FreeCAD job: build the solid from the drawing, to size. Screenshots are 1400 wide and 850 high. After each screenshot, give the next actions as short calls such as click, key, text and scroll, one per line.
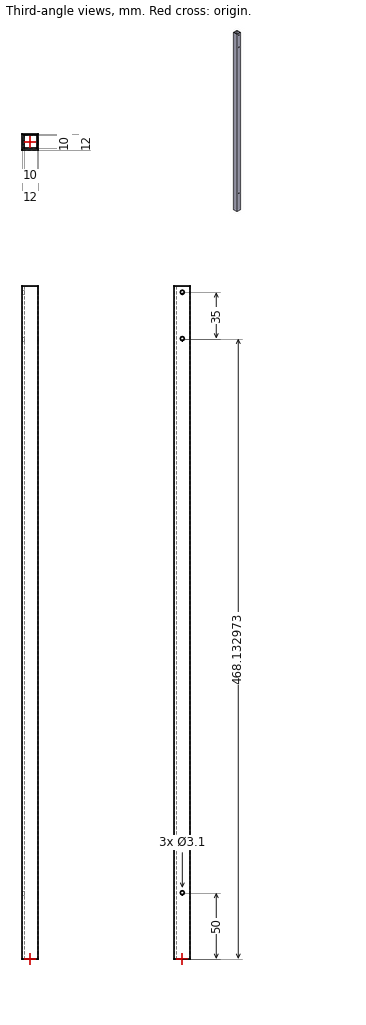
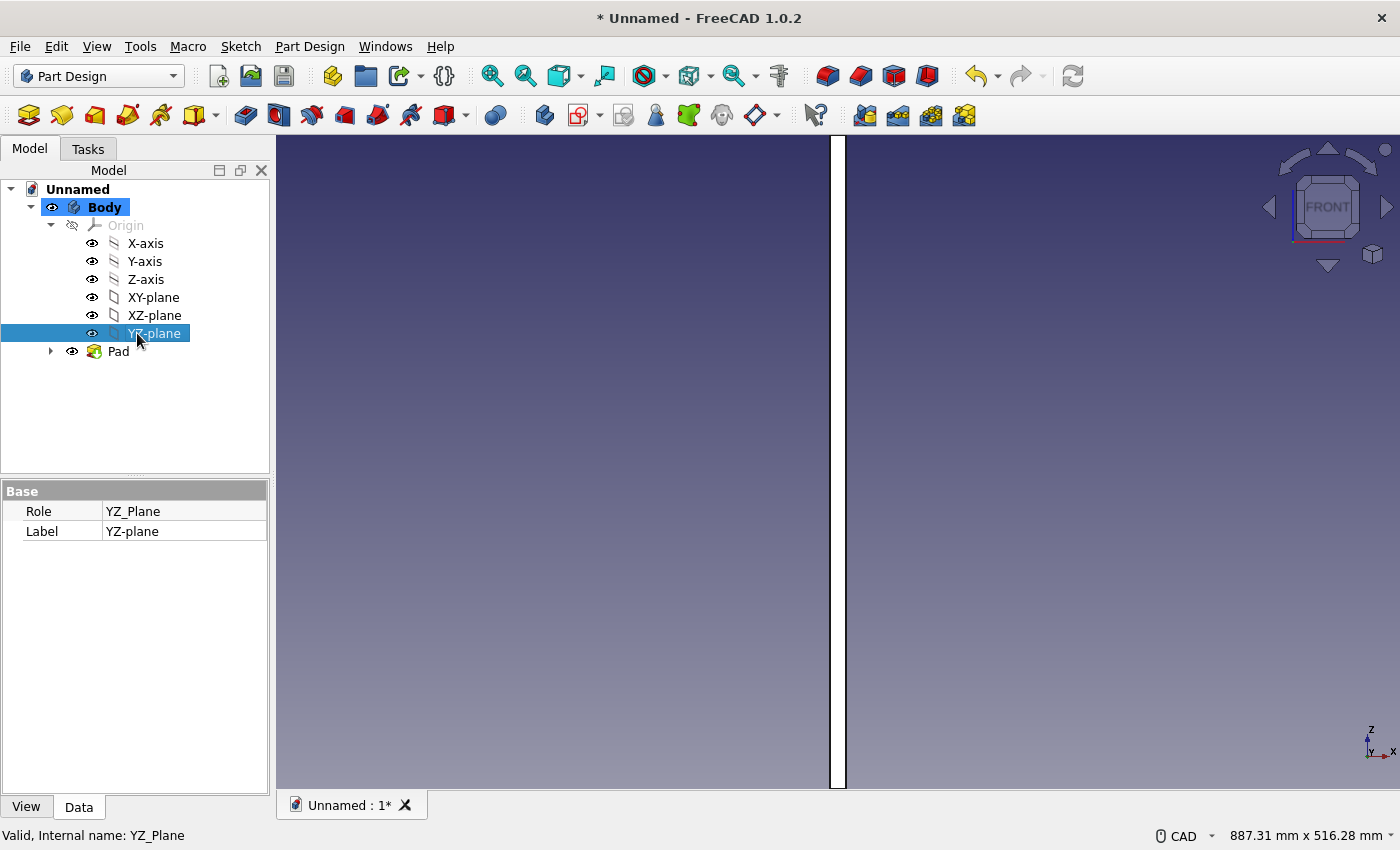
click(754, 116)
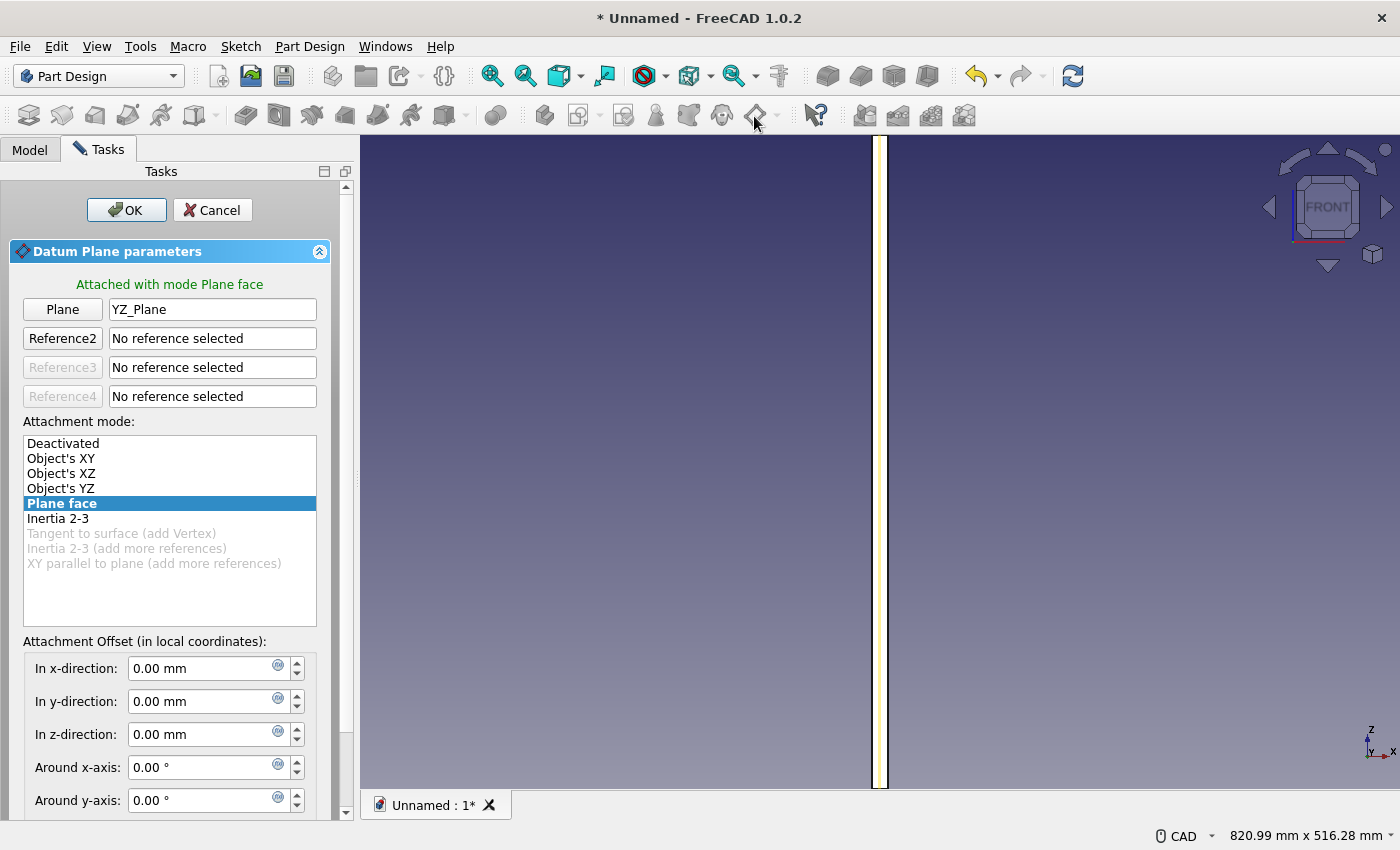
triple_click(210, 734)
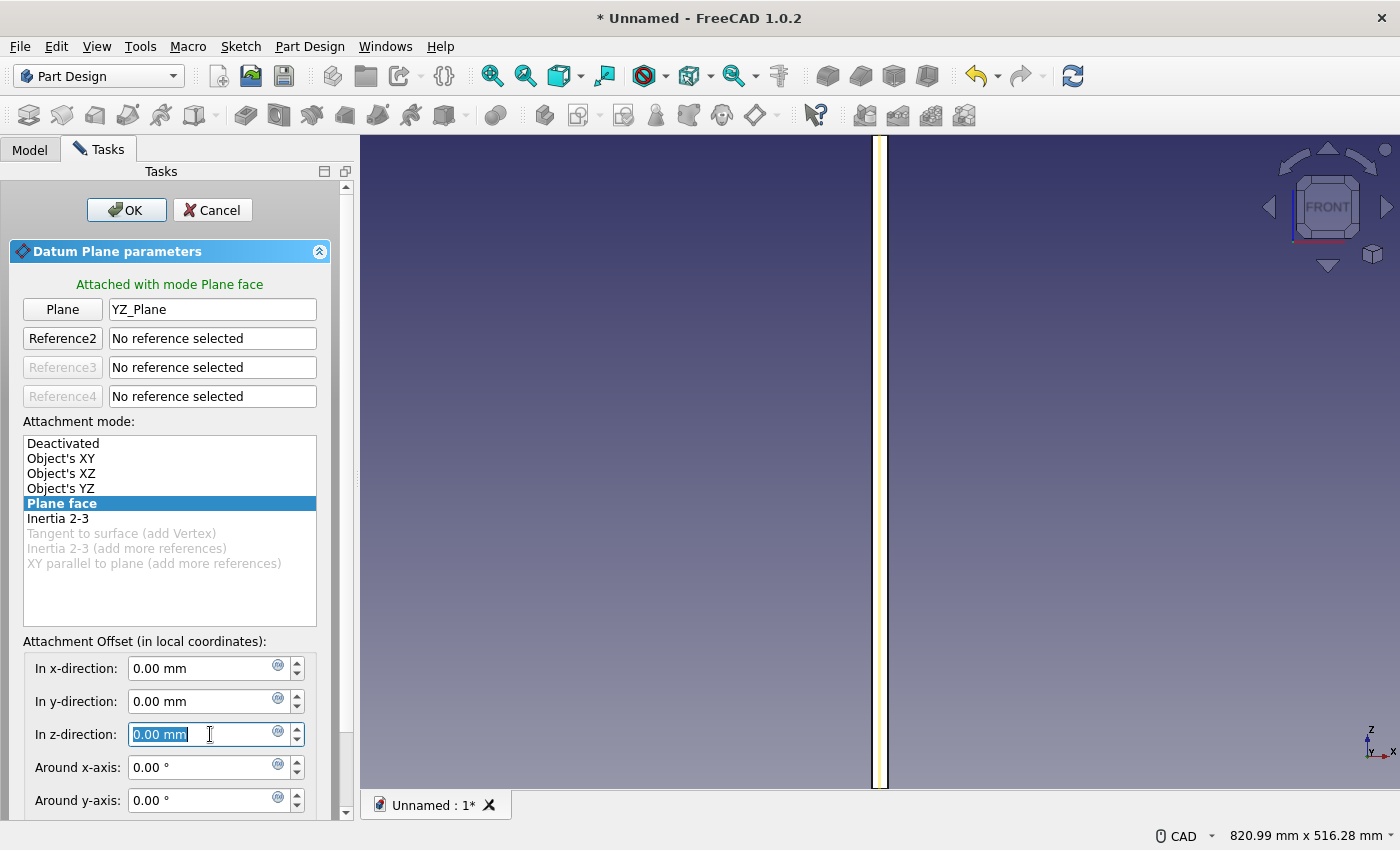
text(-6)
key(Tab)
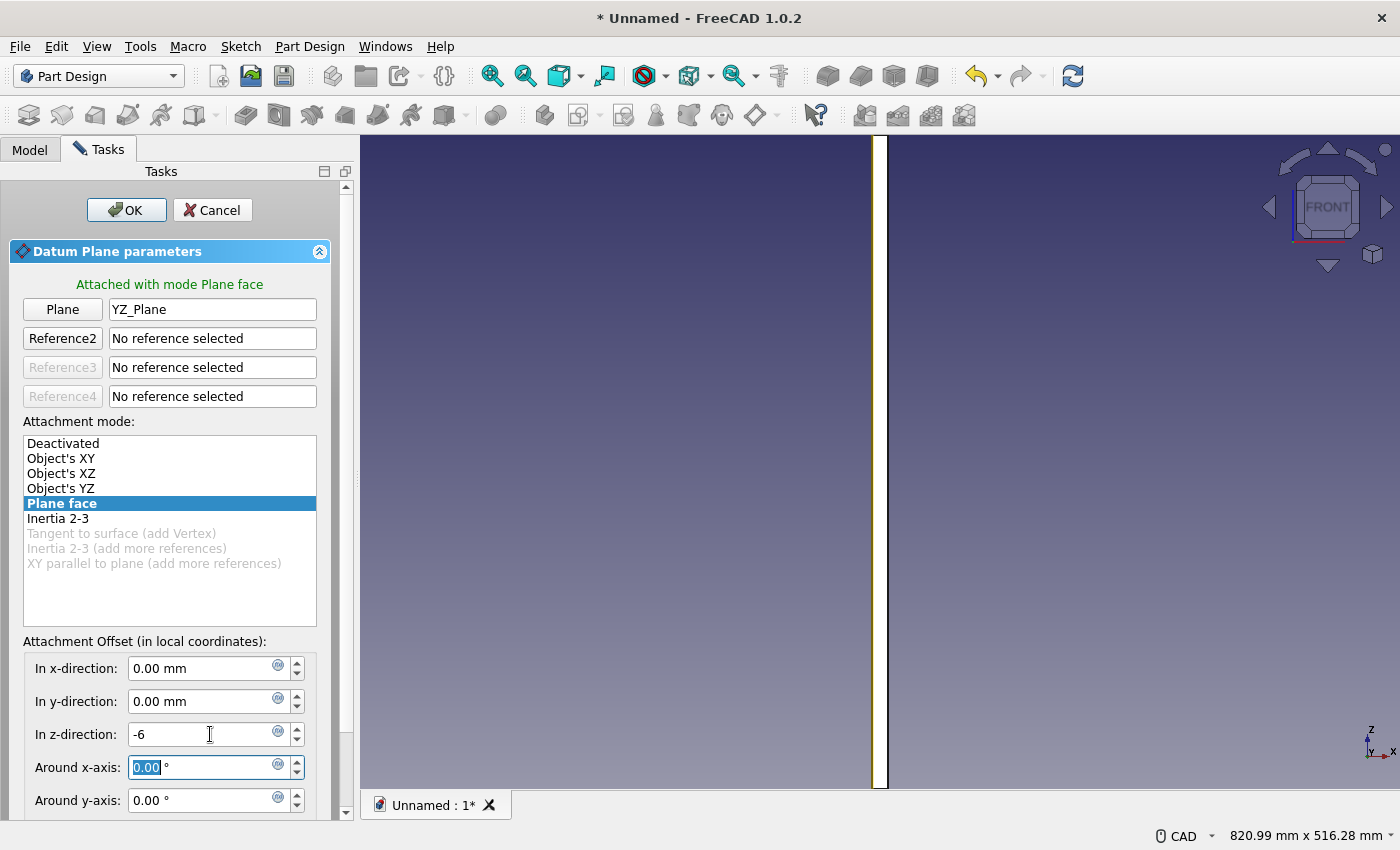
click(127, 210)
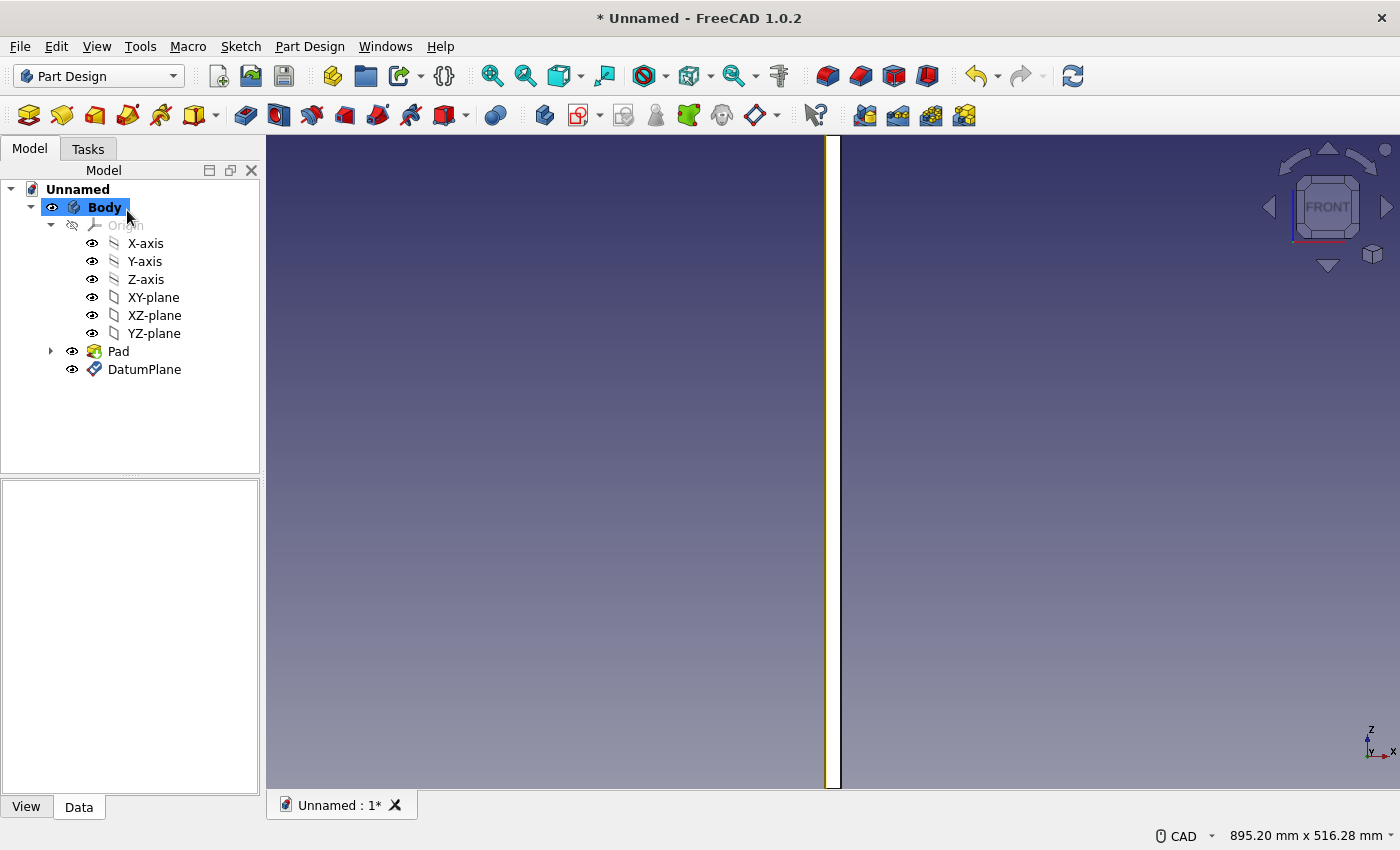
click(117, 369)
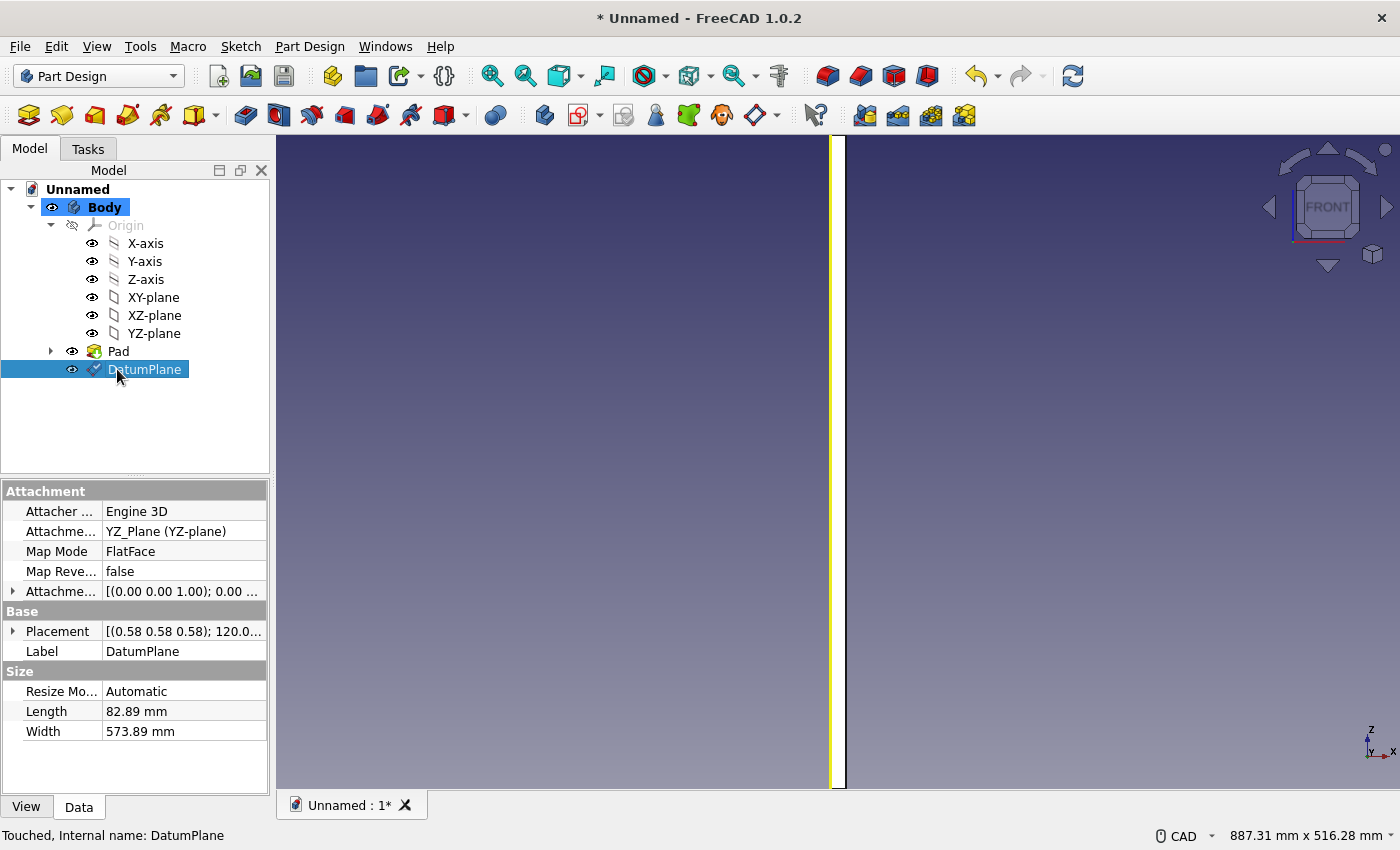
click(578, 116)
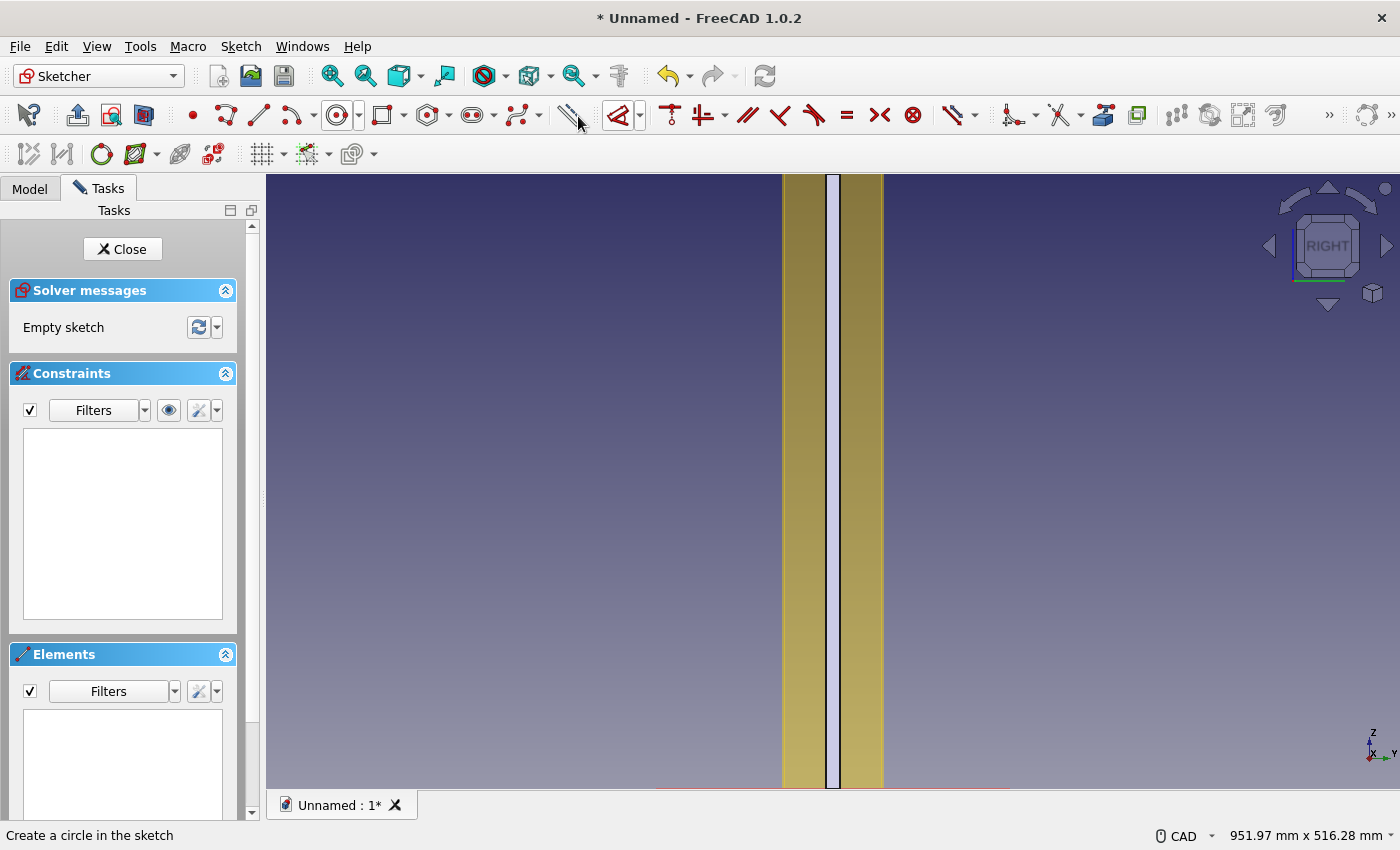
click(144, 116)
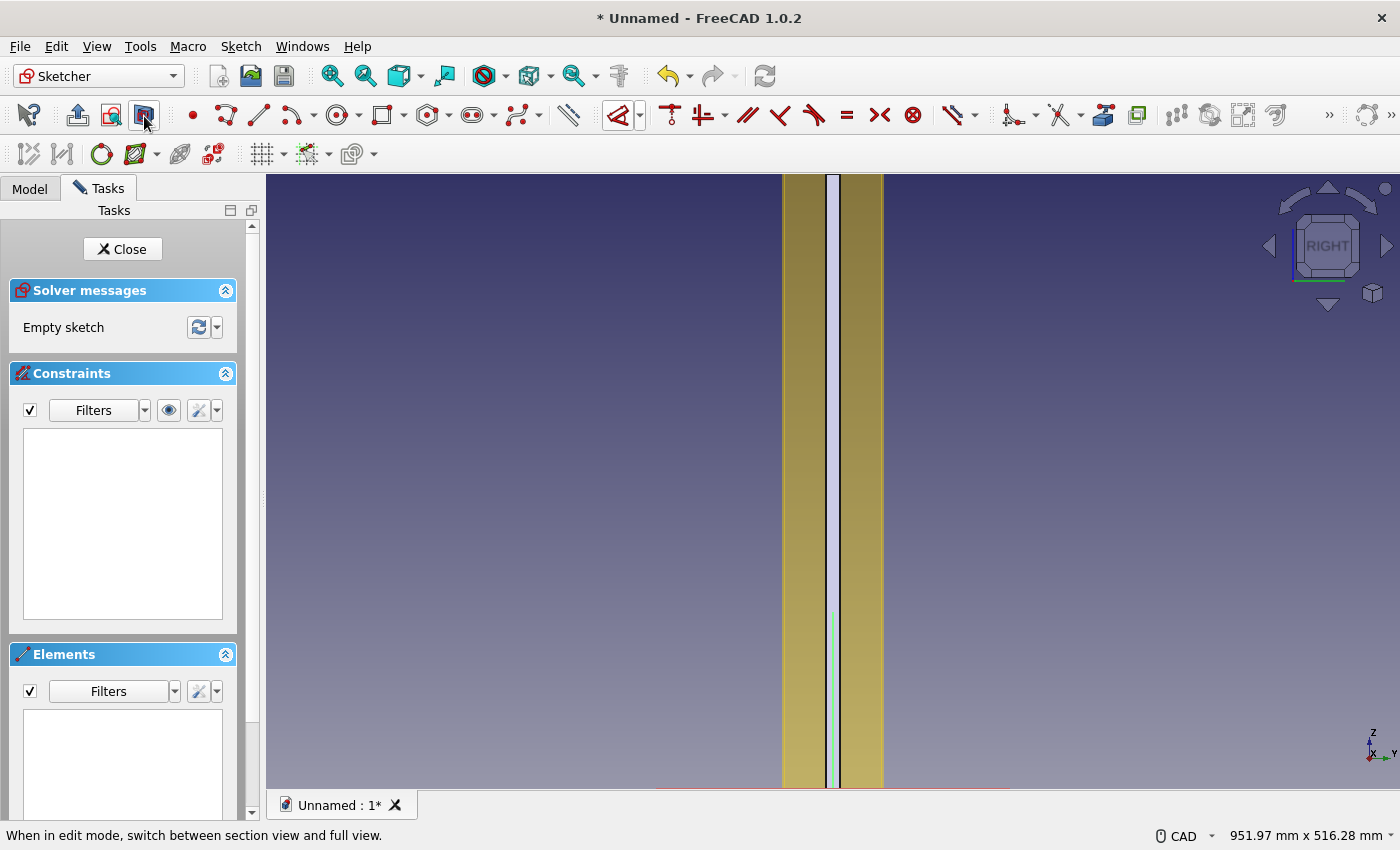
scroll(625, 468, down, 2)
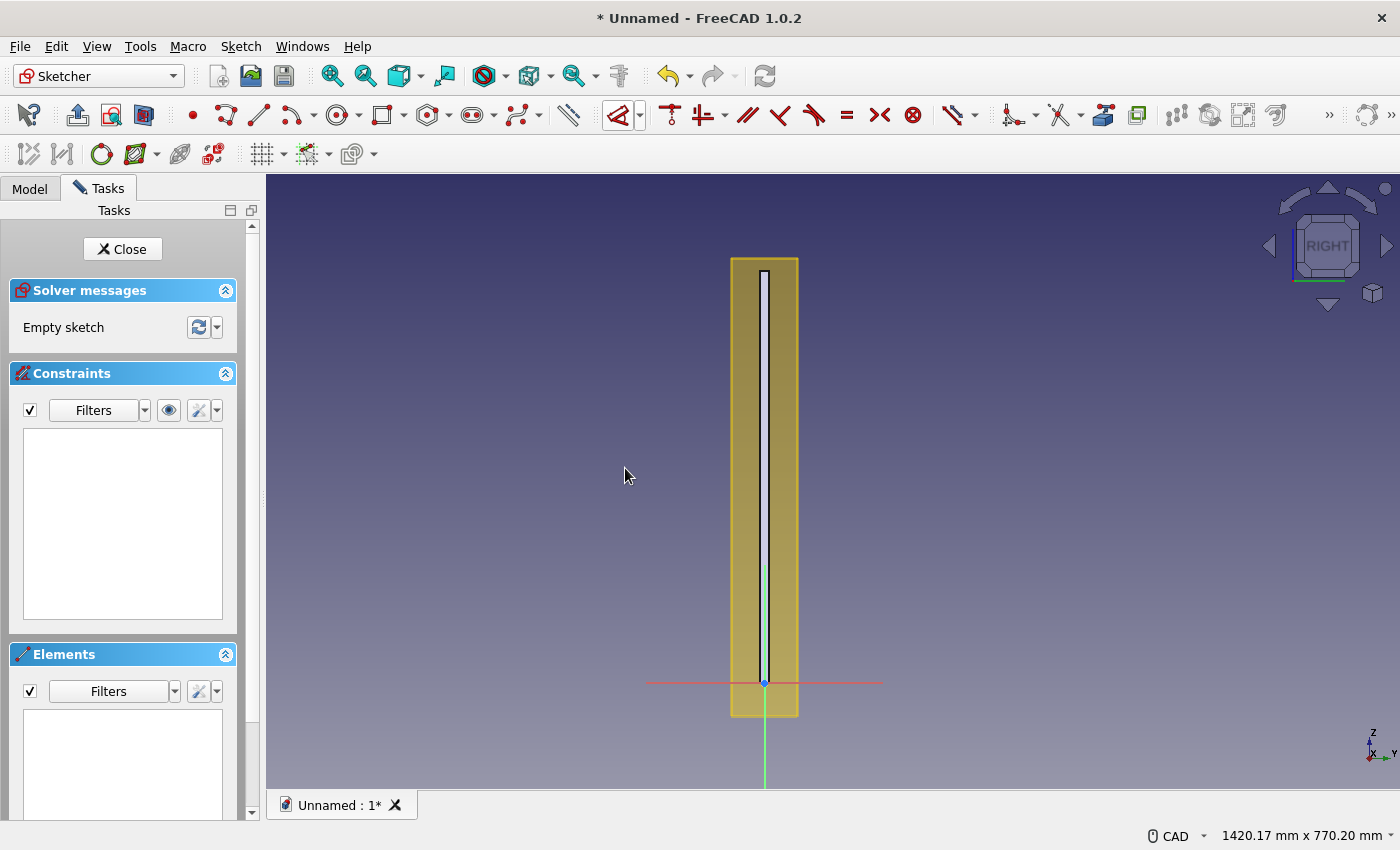
click(336, 116)